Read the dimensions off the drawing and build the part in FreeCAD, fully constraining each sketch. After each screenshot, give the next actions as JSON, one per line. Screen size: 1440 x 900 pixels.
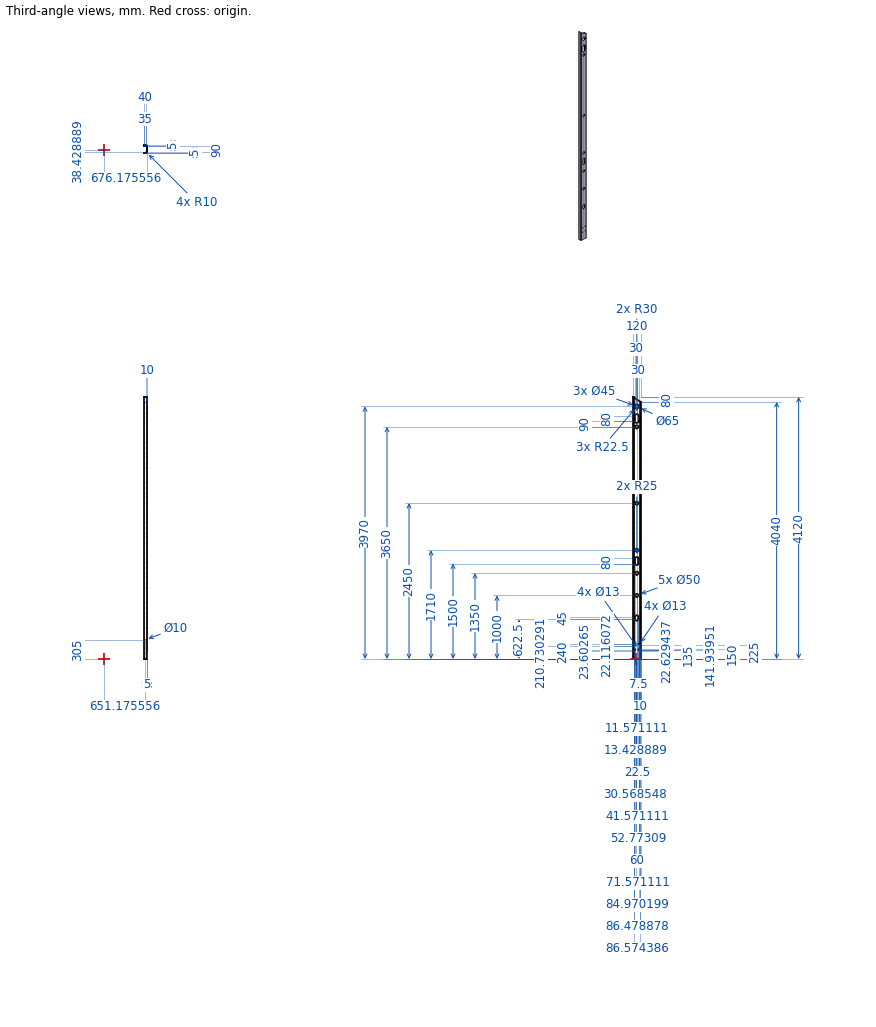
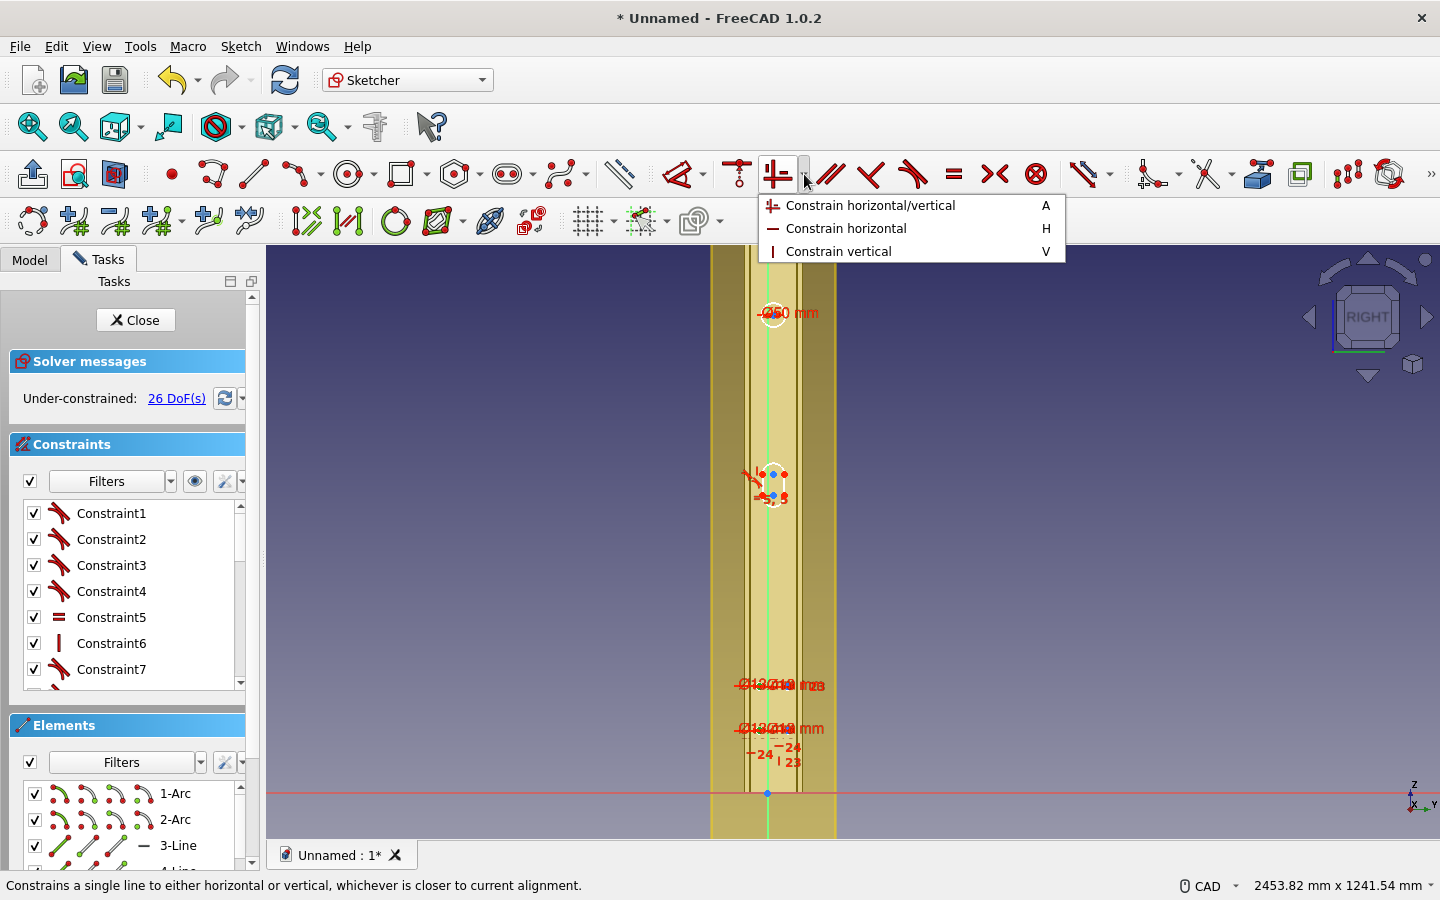
{"action": "left_click", "coordinate": [912, 252]}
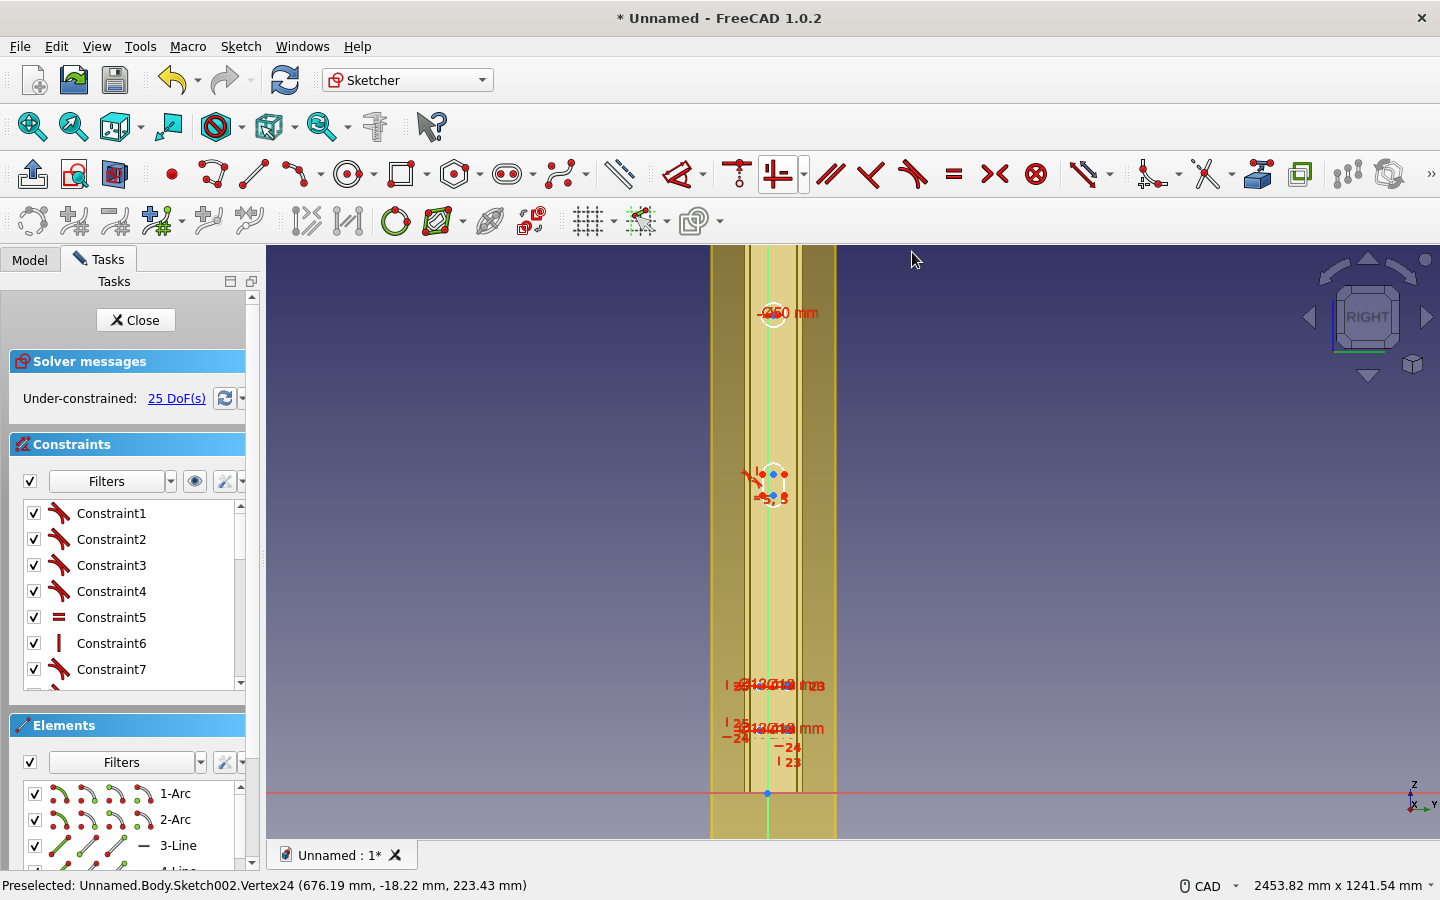
{"action": "left_click", "coordinate": [788, 687]}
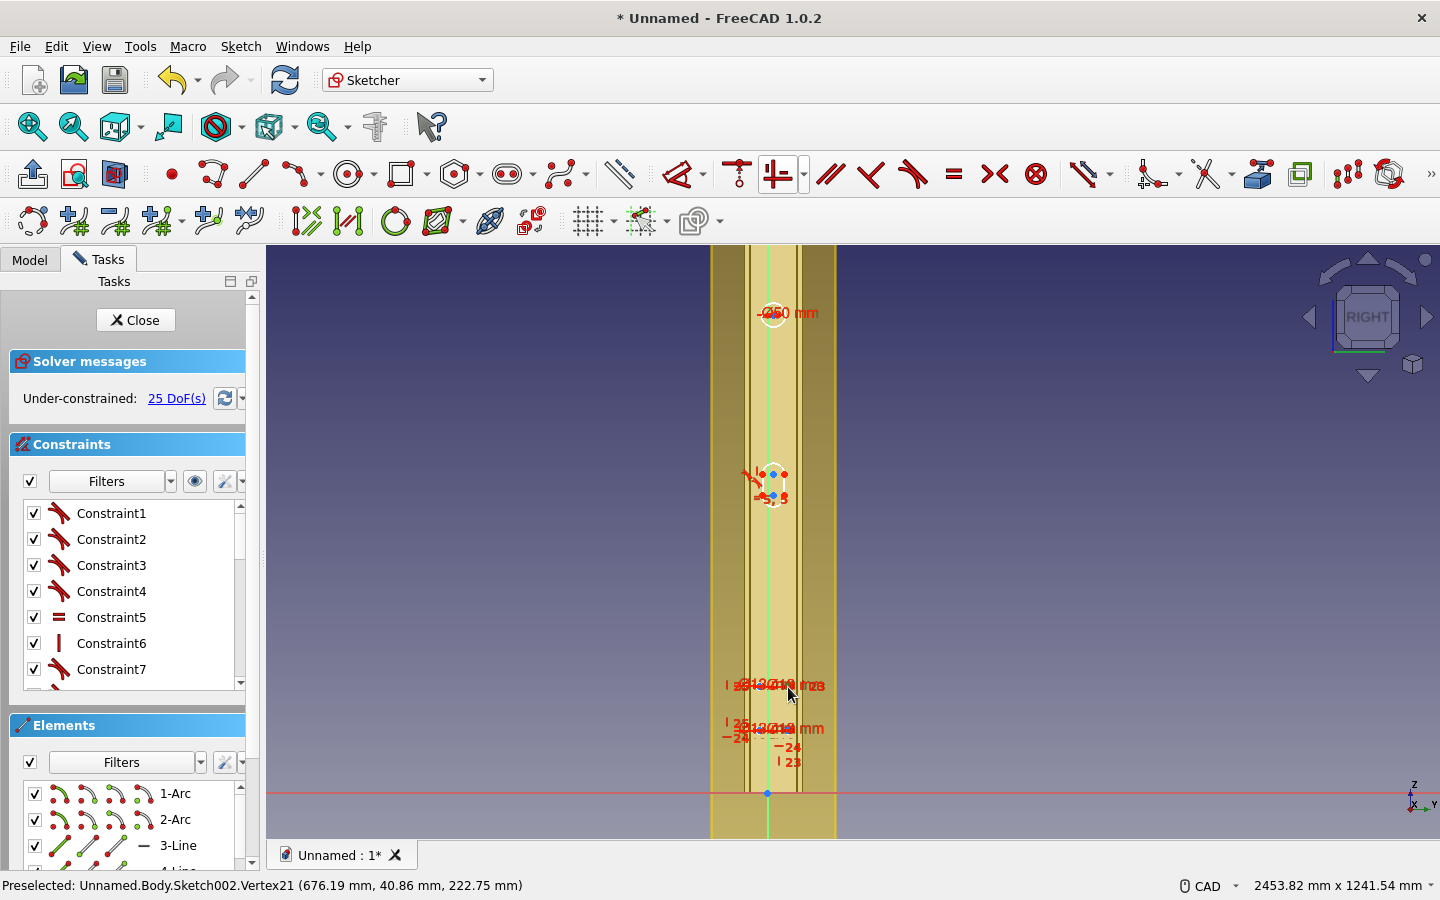
{"action": "left_click", "coordinate": [759, 686]}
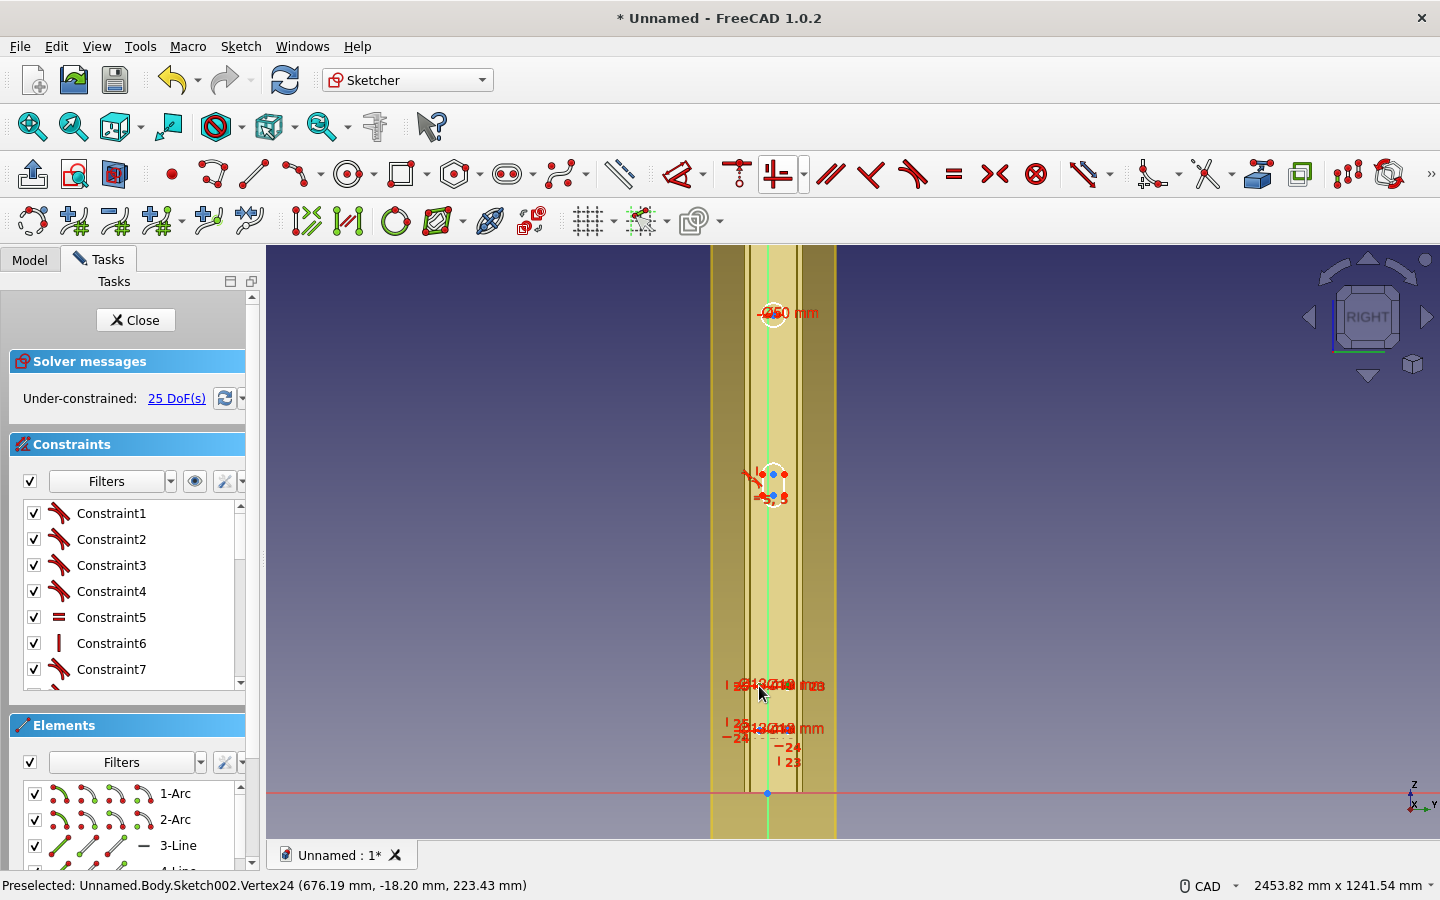
{"action": "key", "text": "h"}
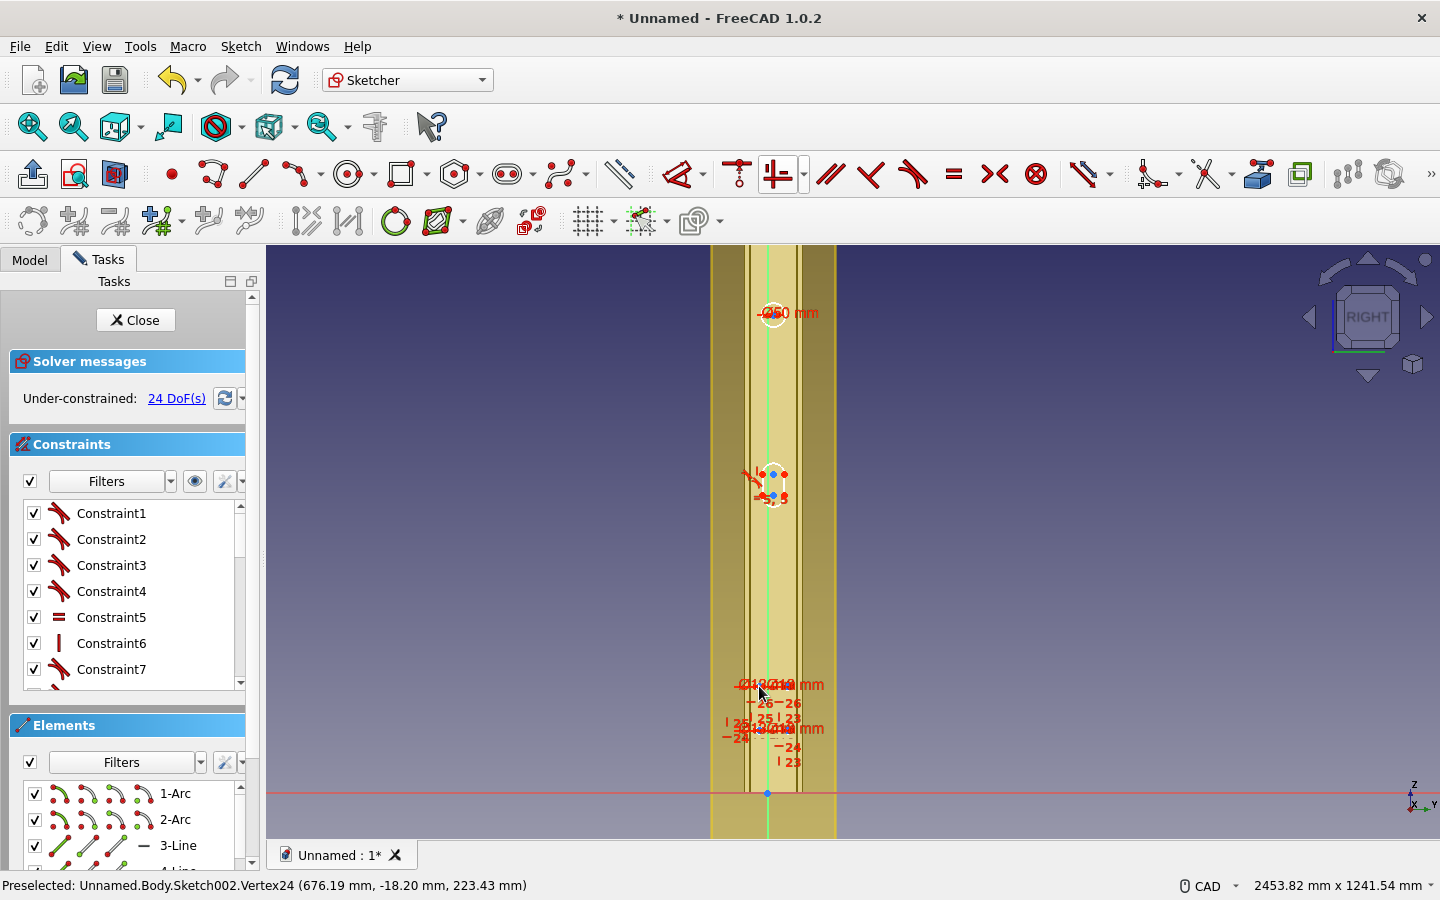
{"action": "scroll", "coordinate": [787, 720], "scroll_direction": "down", "scroll_amount": 8}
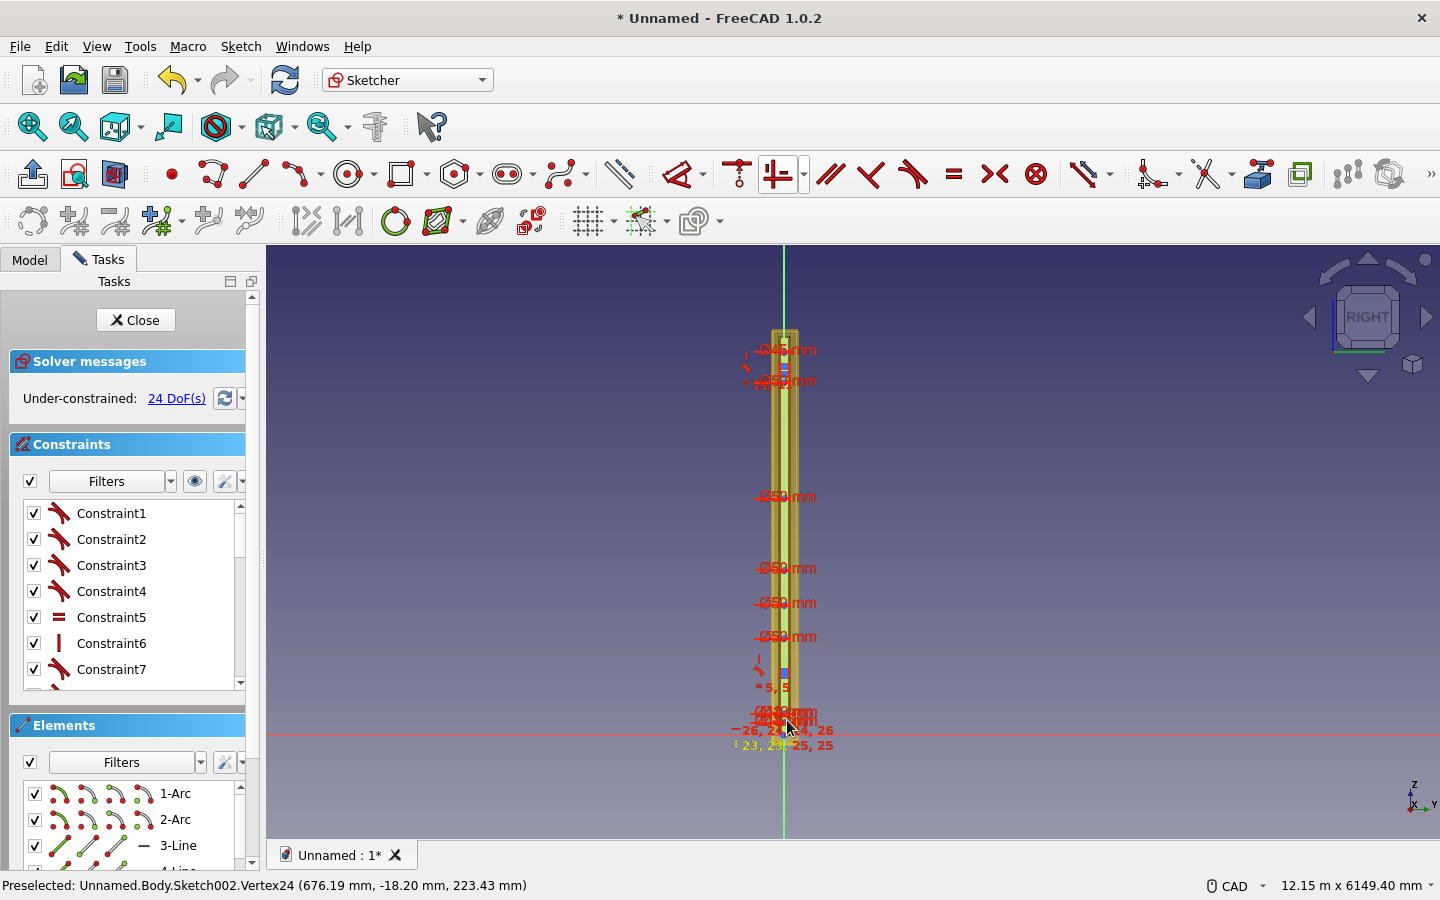
{"action": "left_click", "coordinate": [785, 639]}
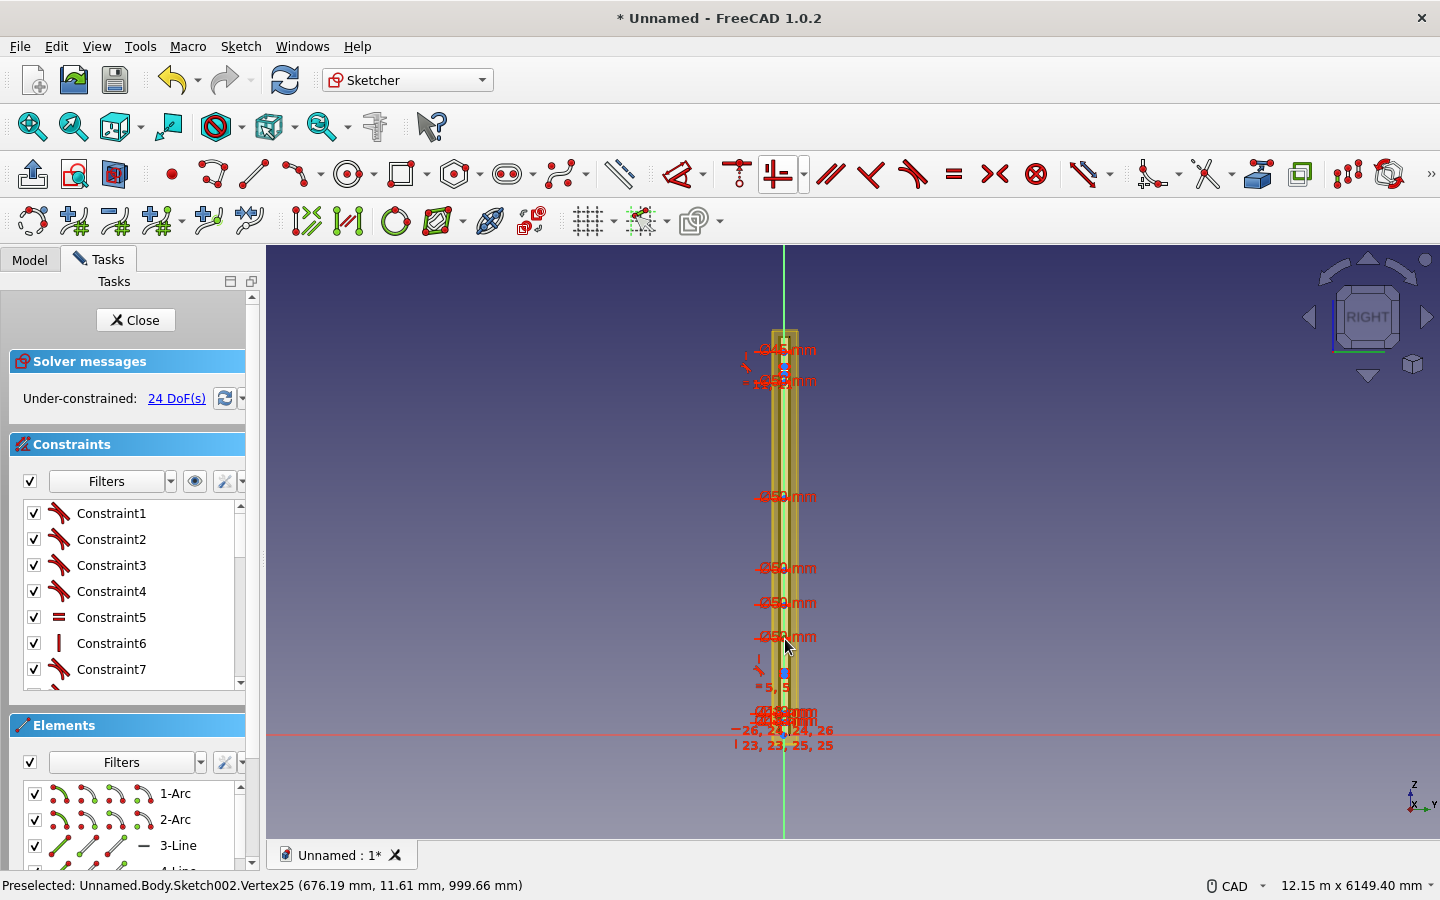
{"action": "left_click", "coordinate": [785, 605]}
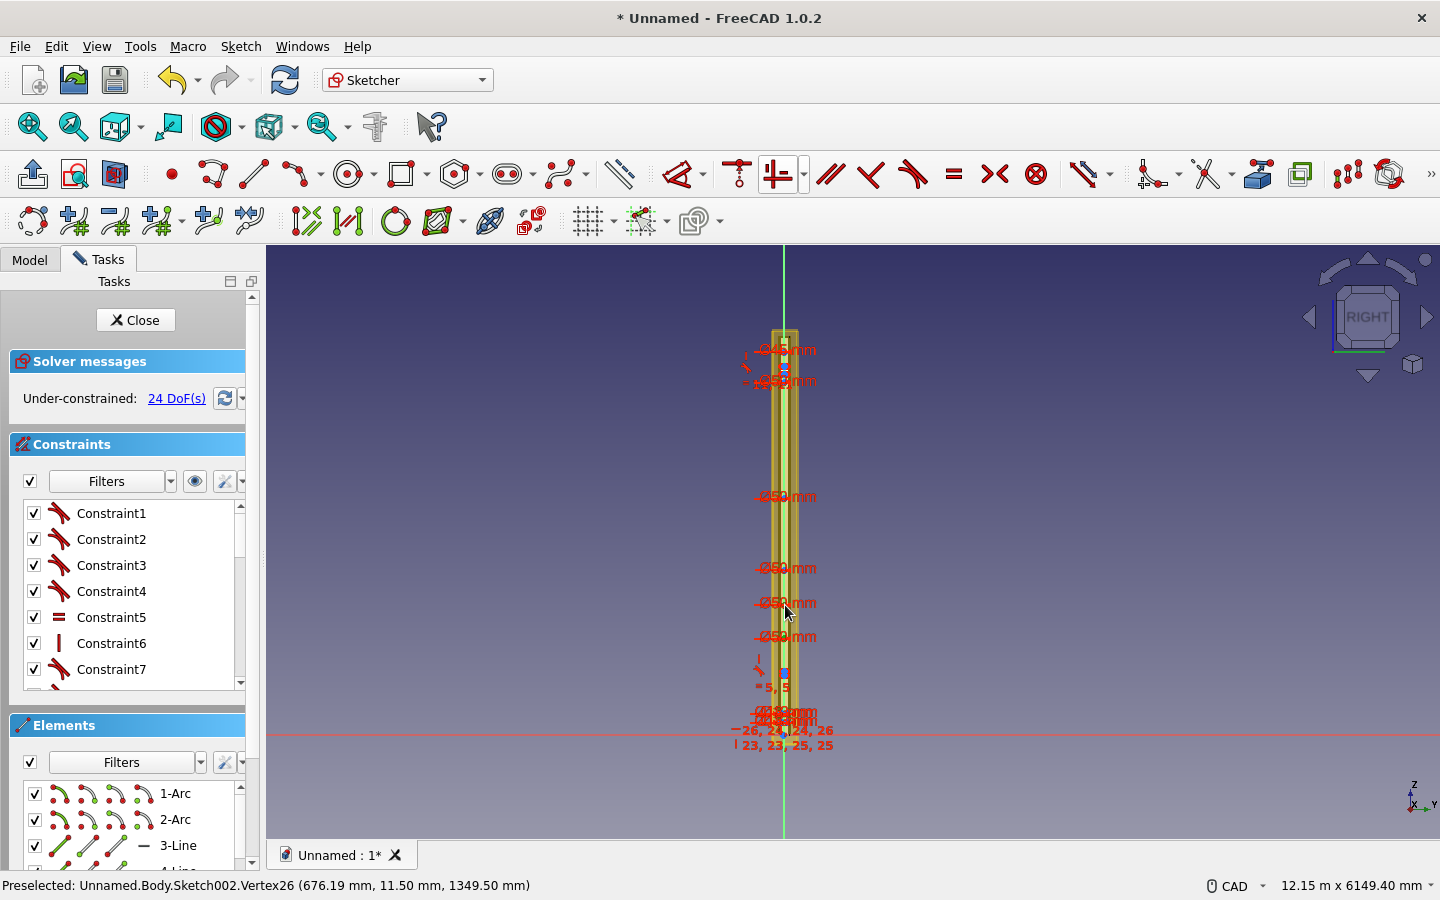
{"action": "key", "text": "v"}